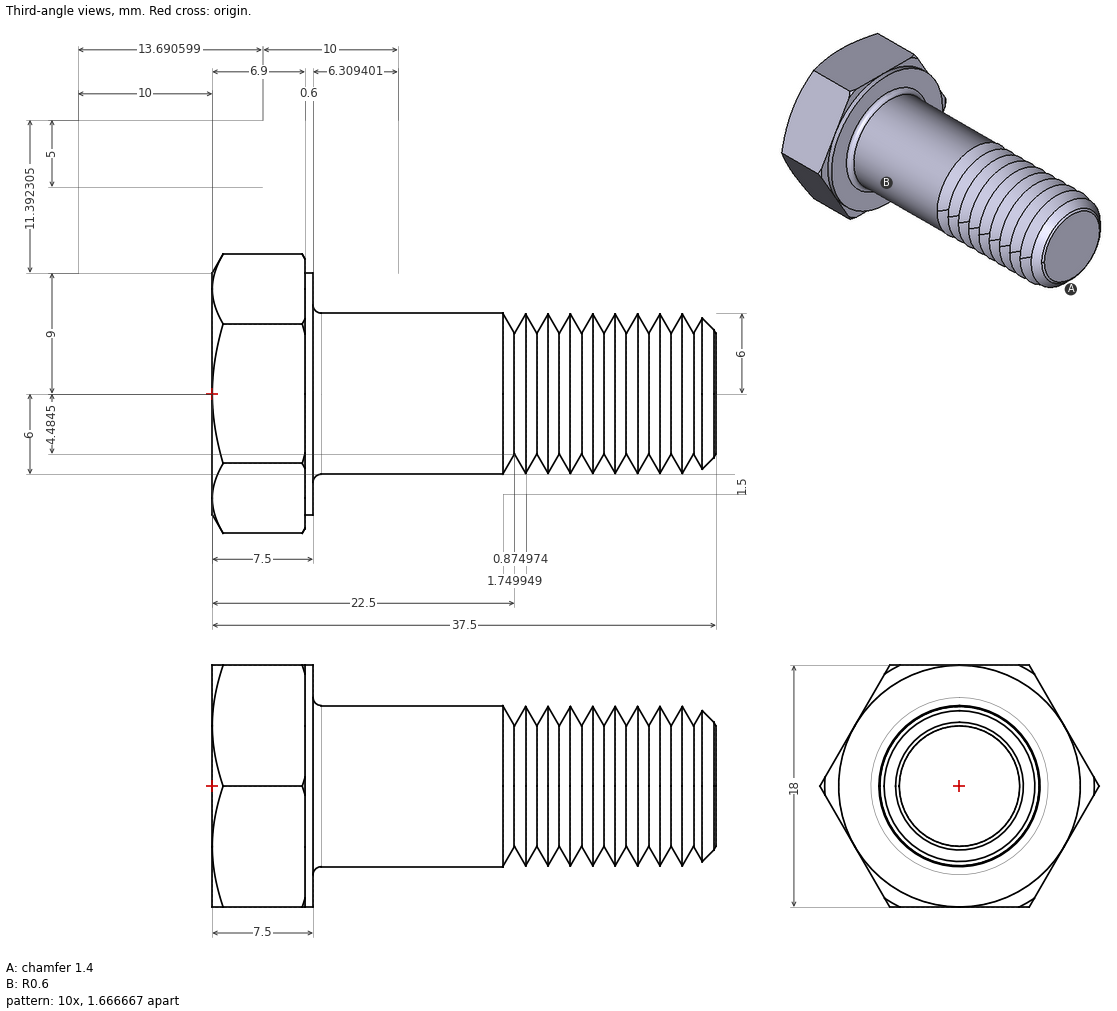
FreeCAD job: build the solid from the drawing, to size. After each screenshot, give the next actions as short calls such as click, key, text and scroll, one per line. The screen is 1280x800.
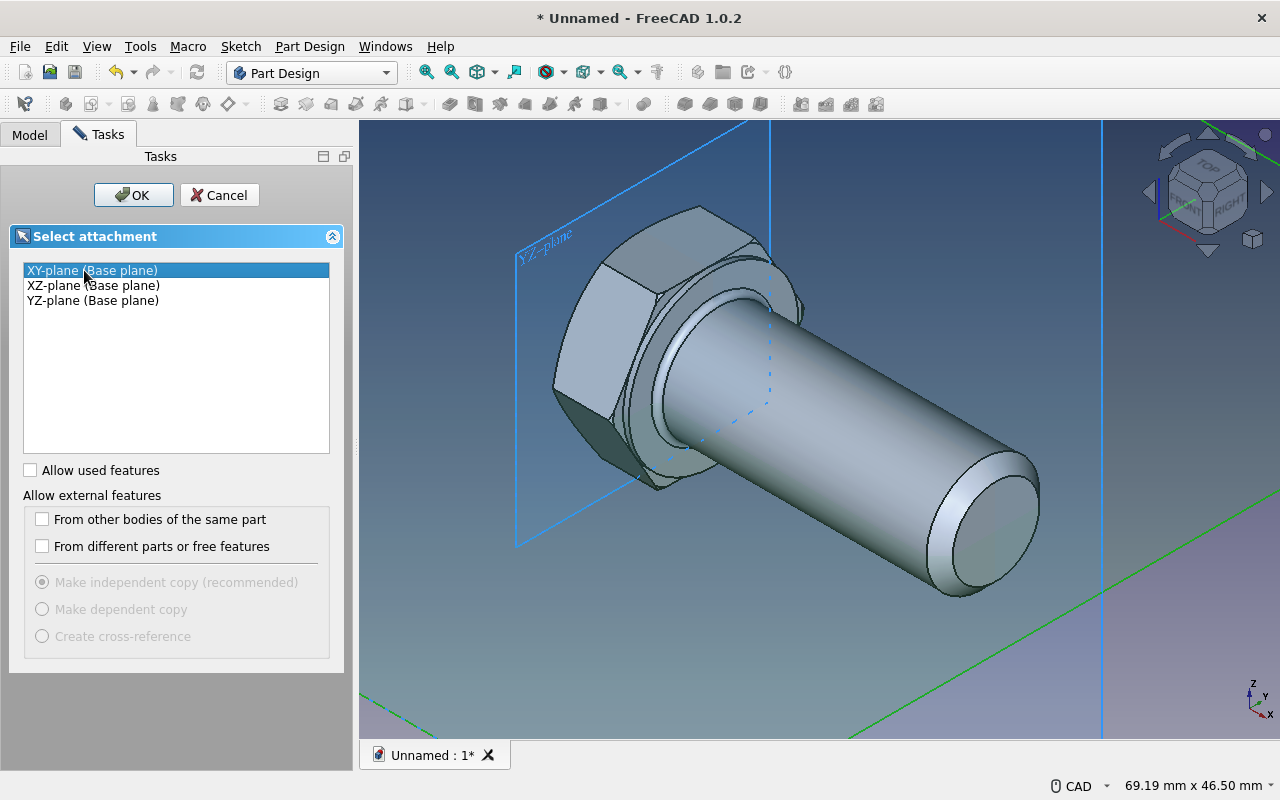
click(134, 195)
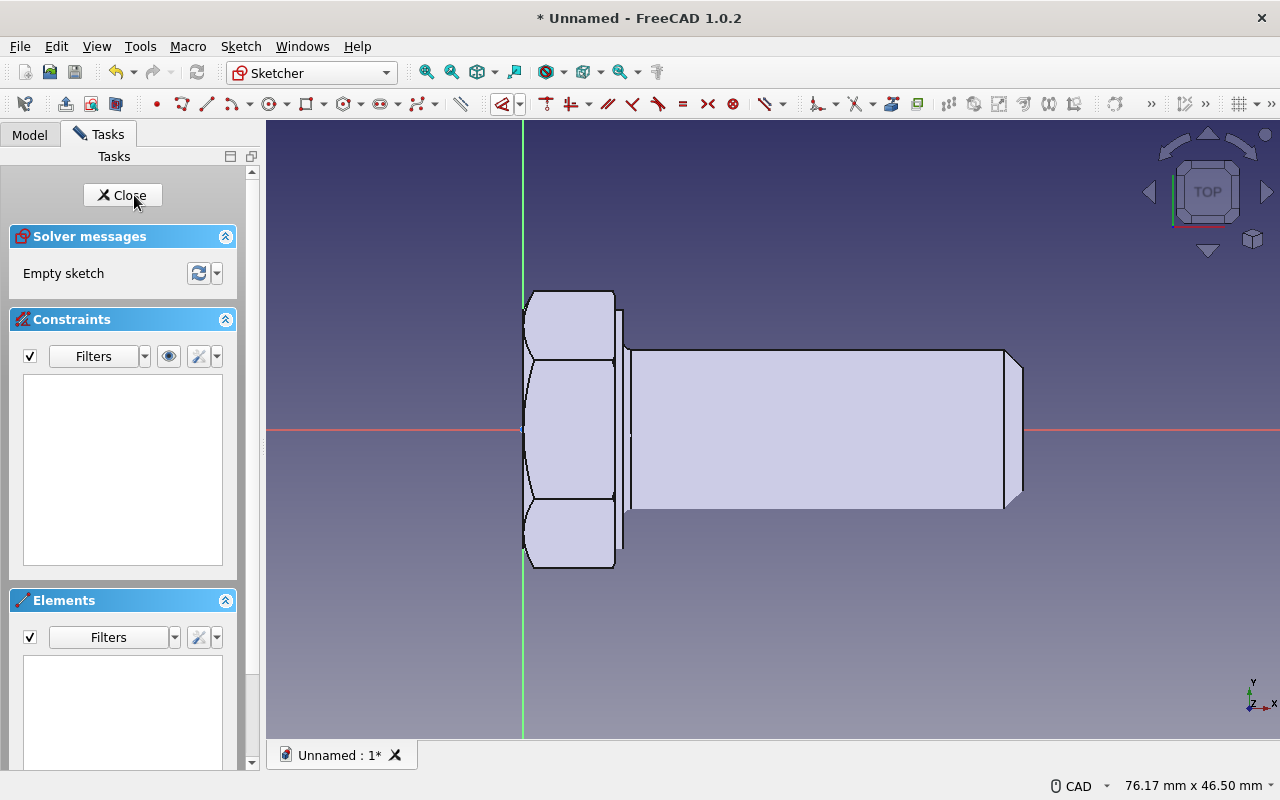
click(116, 104)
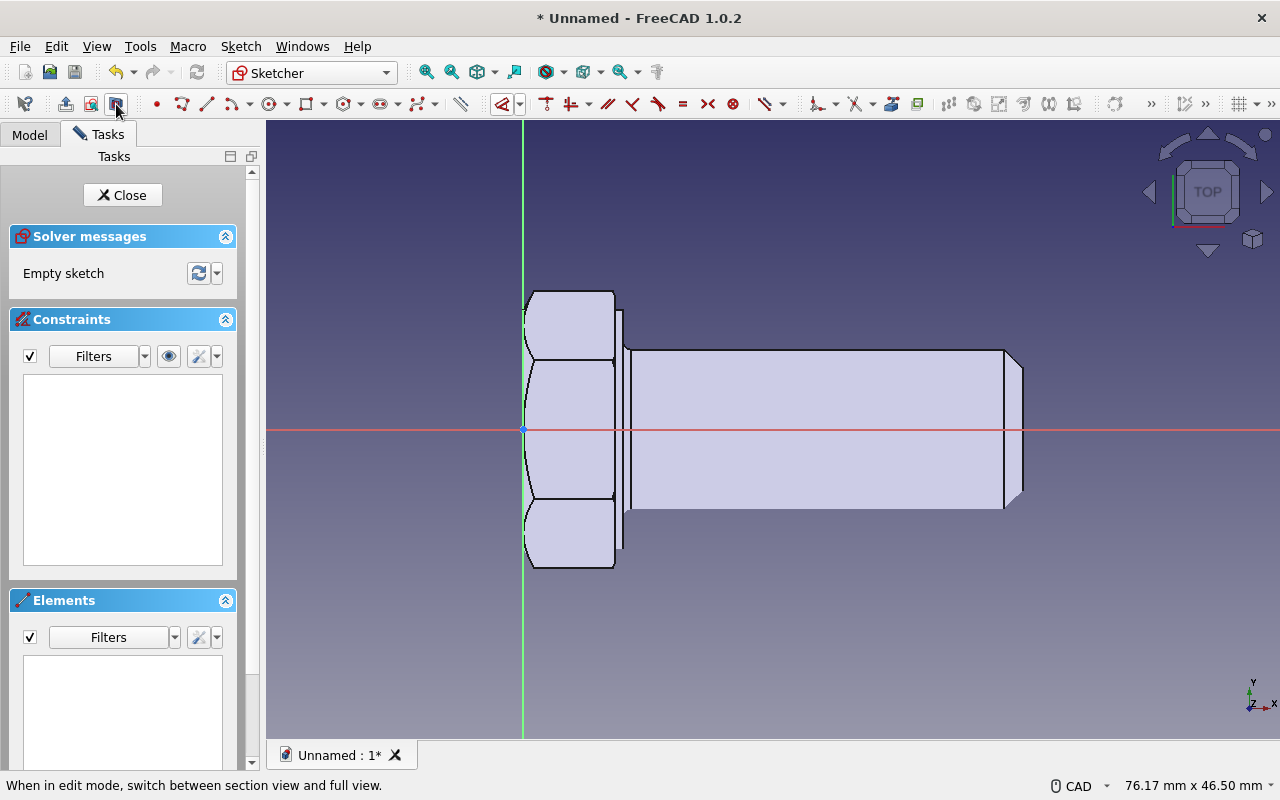
scroll(838, 519, up, 11)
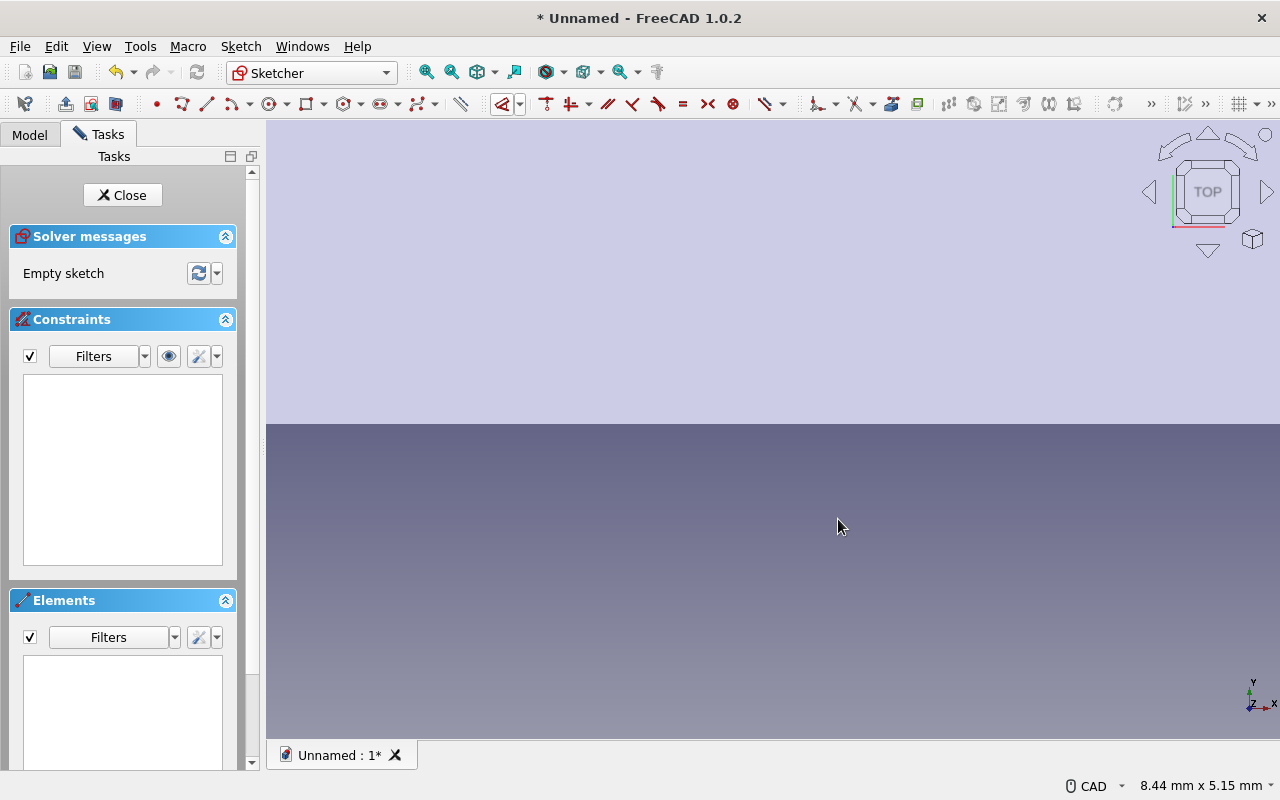
click(182, 104)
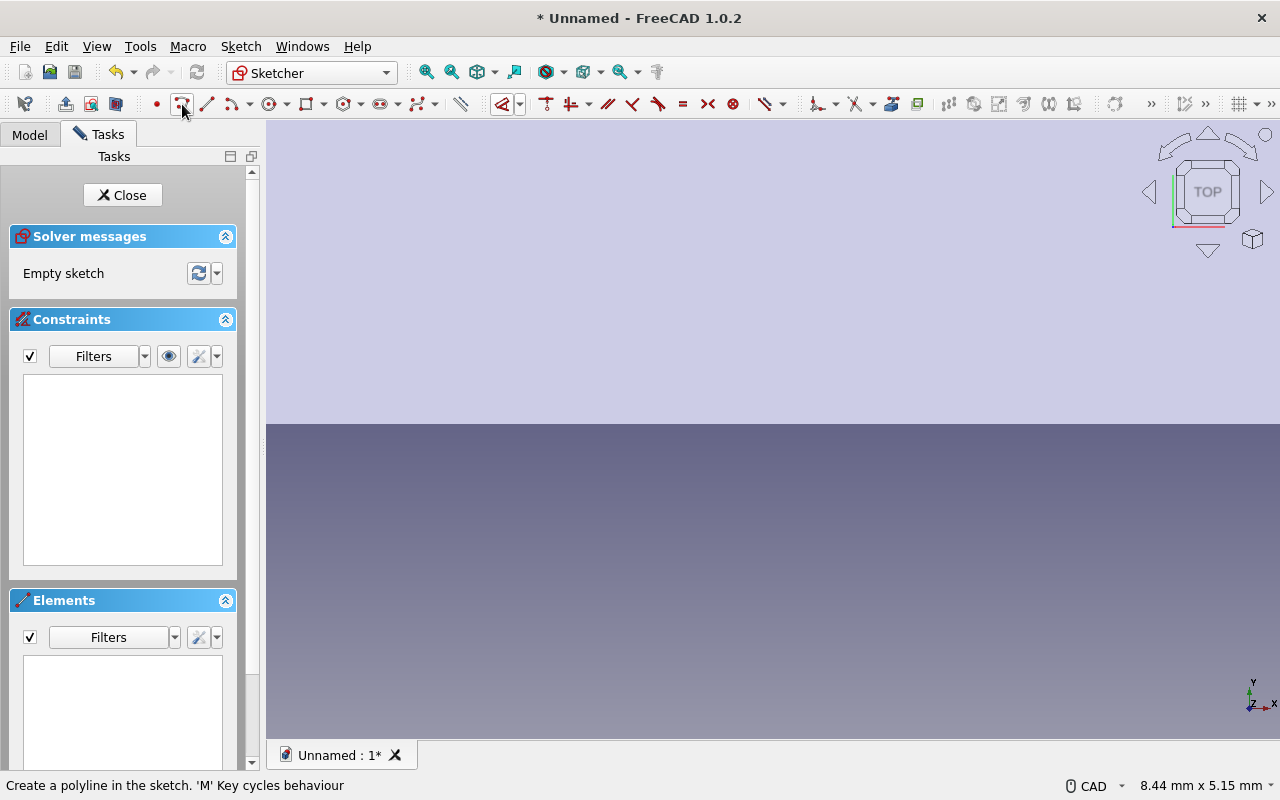
click(592, 427)
click(592, 607)
click(802, 607)
click(802, 427)
click(697, 245)
click(592, 428)
key(Escape)
key(Escape)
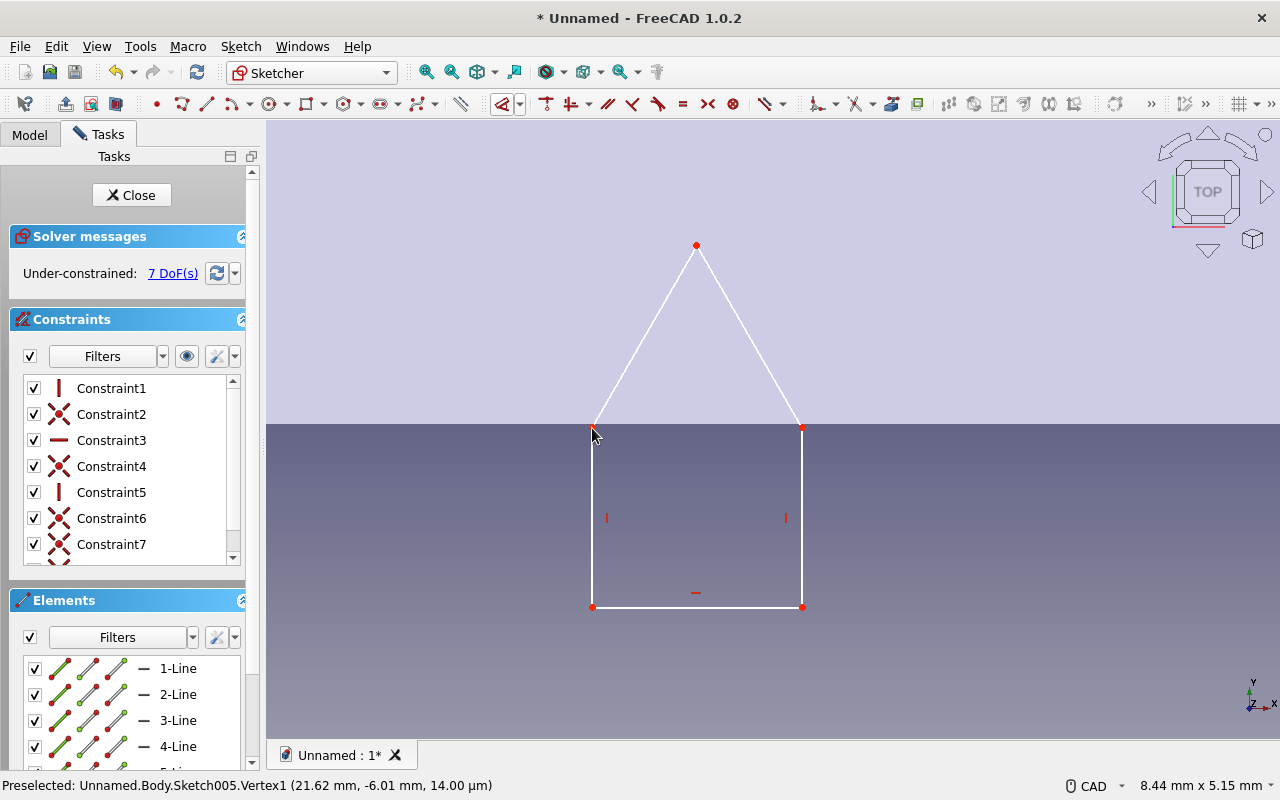
click(592, 428)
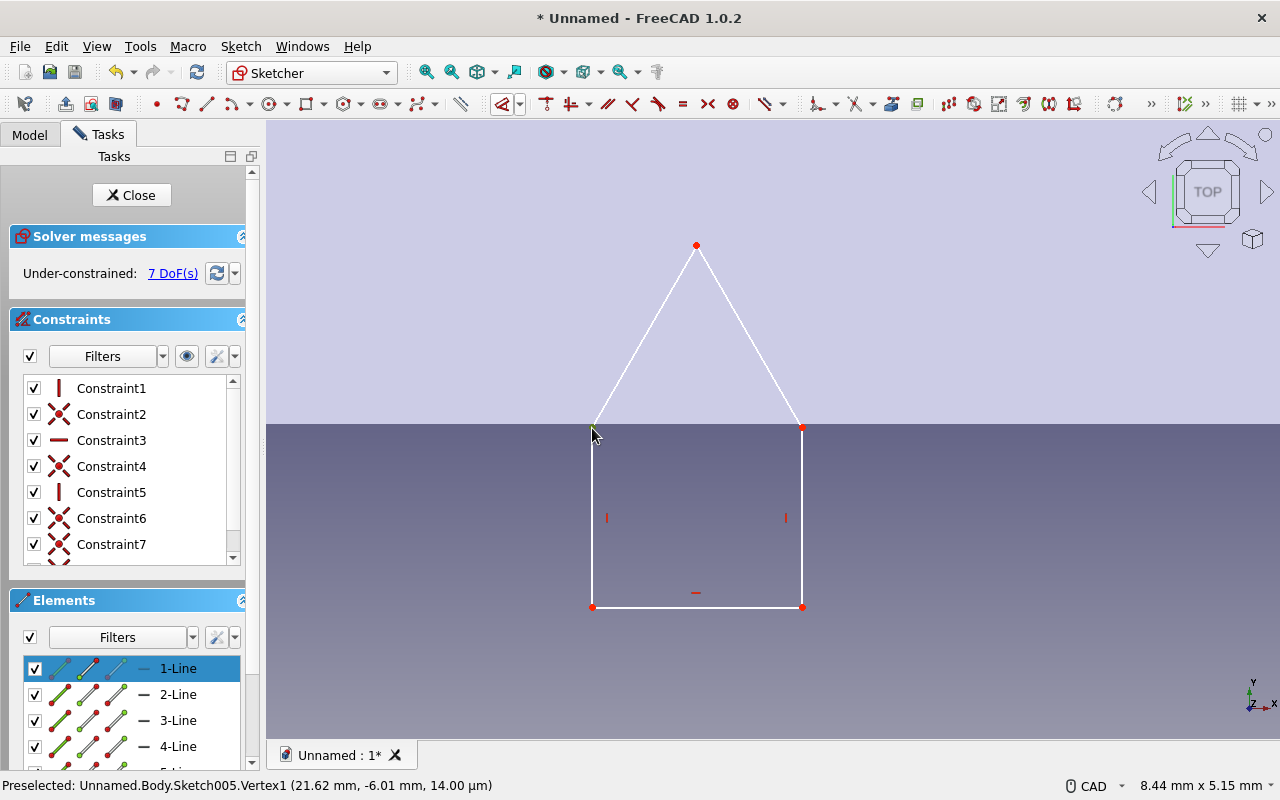
key(i)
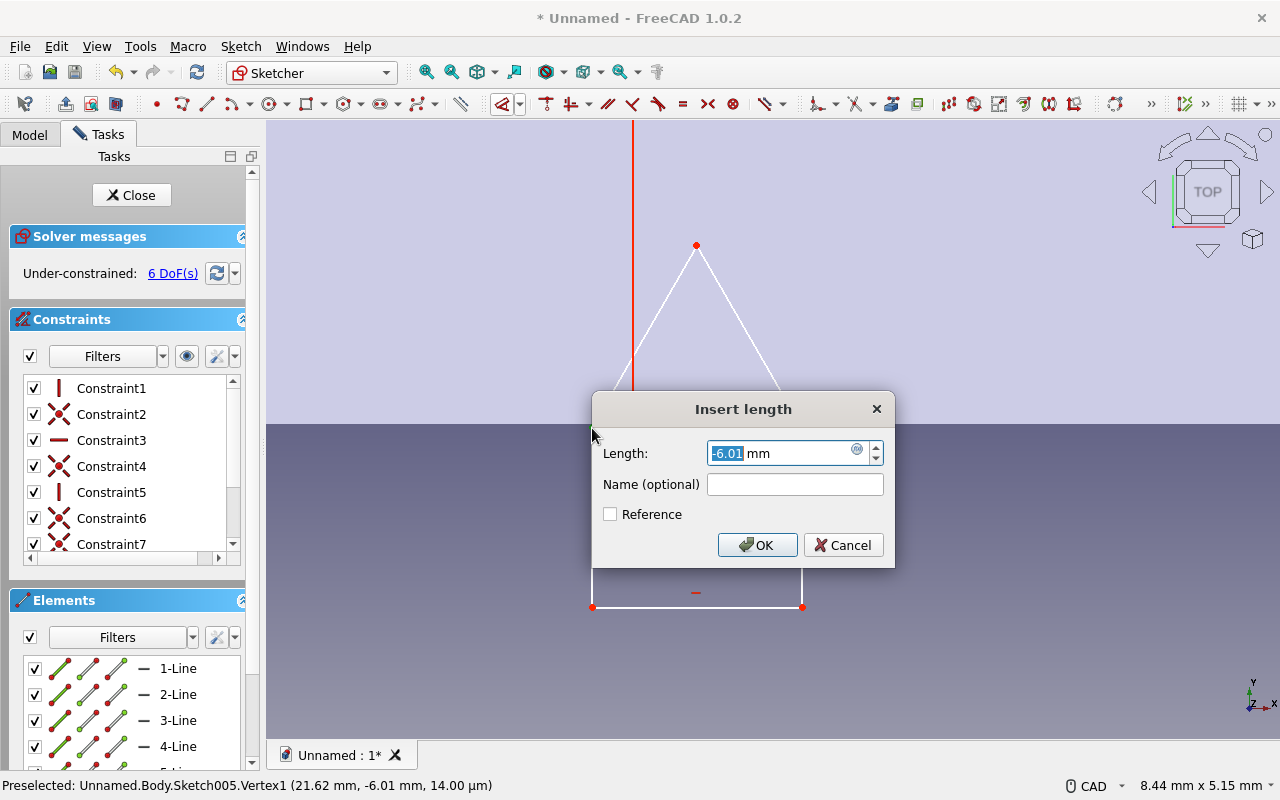
text(-6)
key(Return)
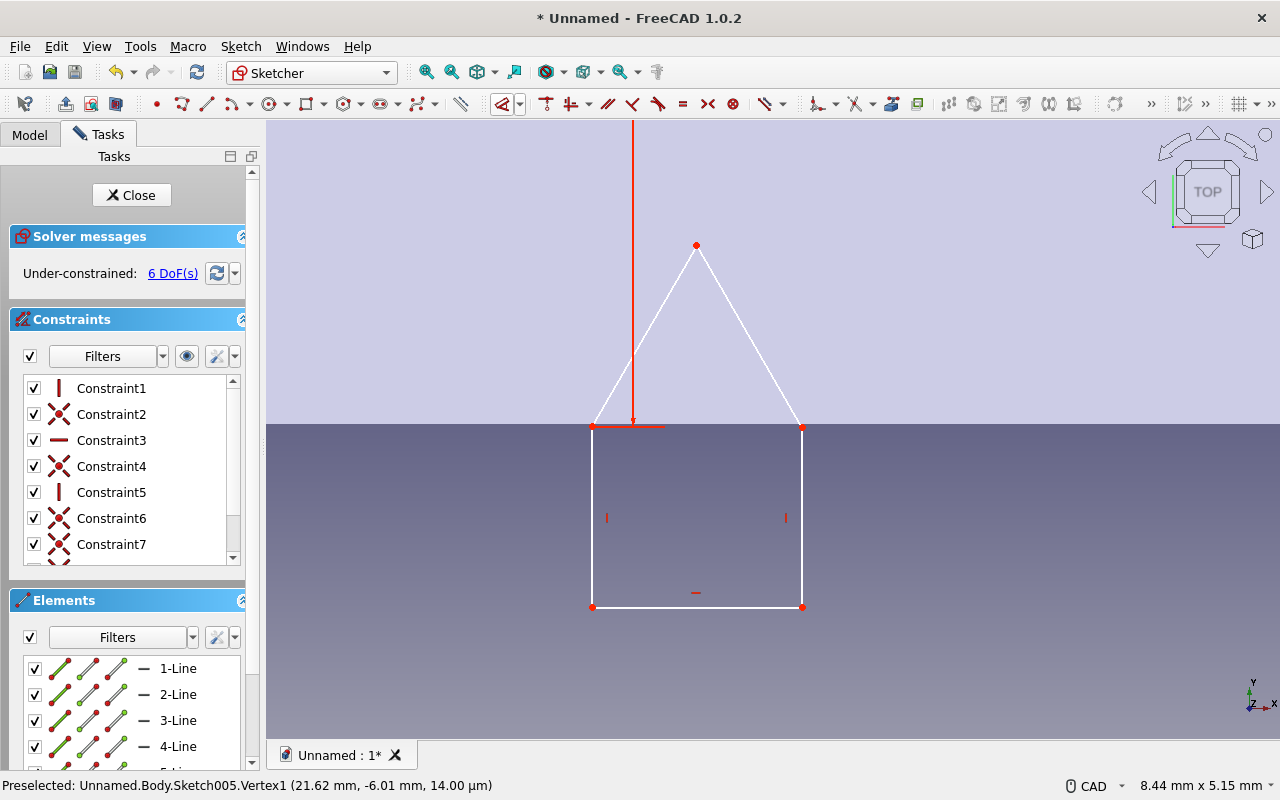
click(802, 428)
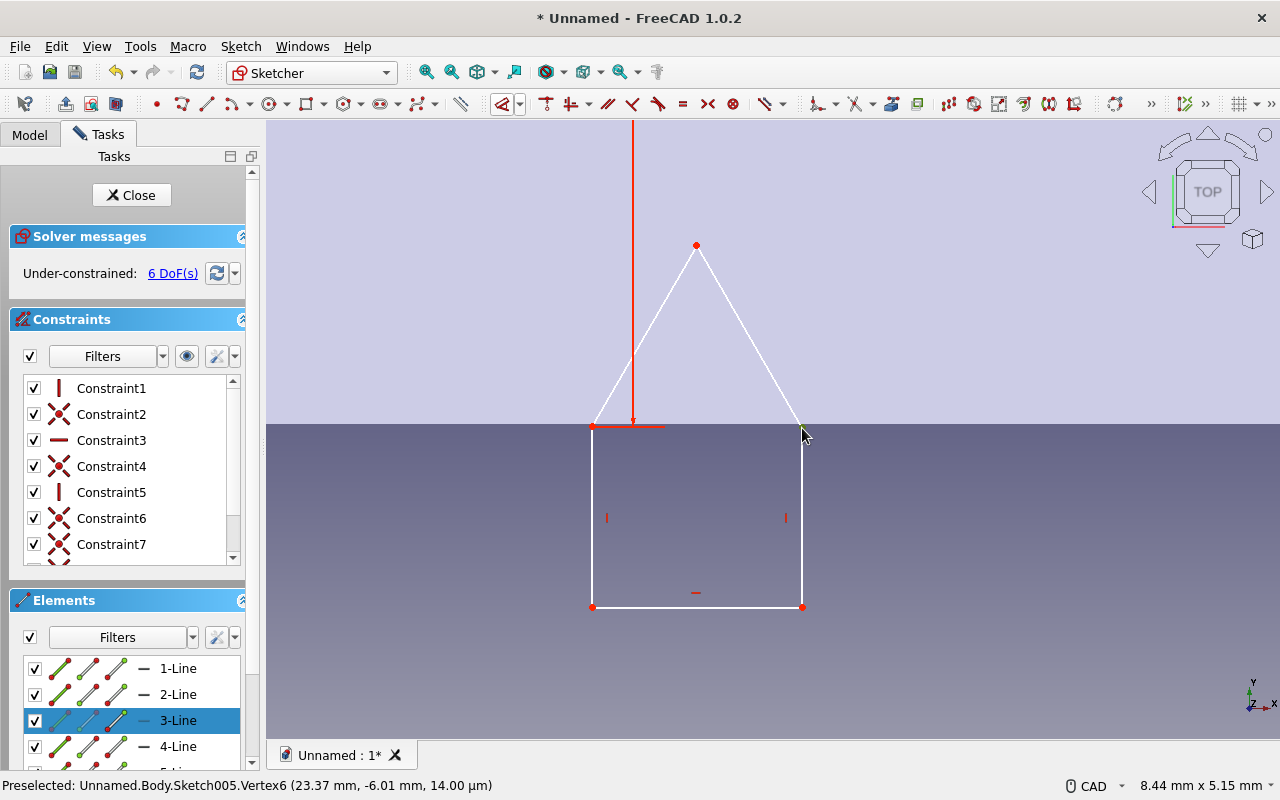
click(520, 104)